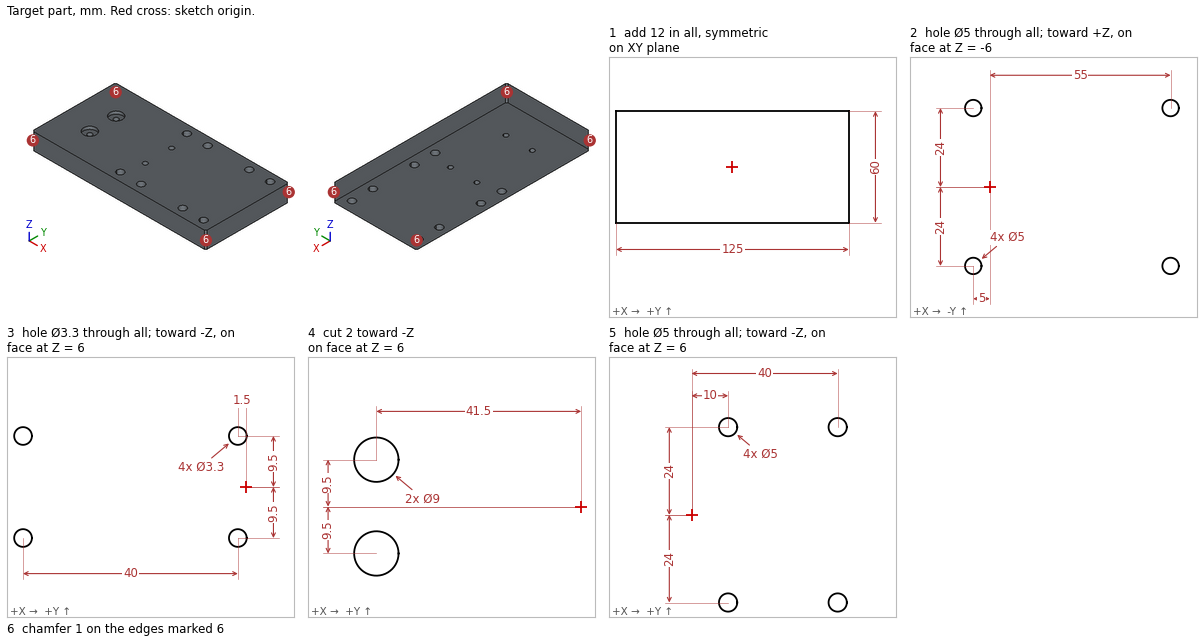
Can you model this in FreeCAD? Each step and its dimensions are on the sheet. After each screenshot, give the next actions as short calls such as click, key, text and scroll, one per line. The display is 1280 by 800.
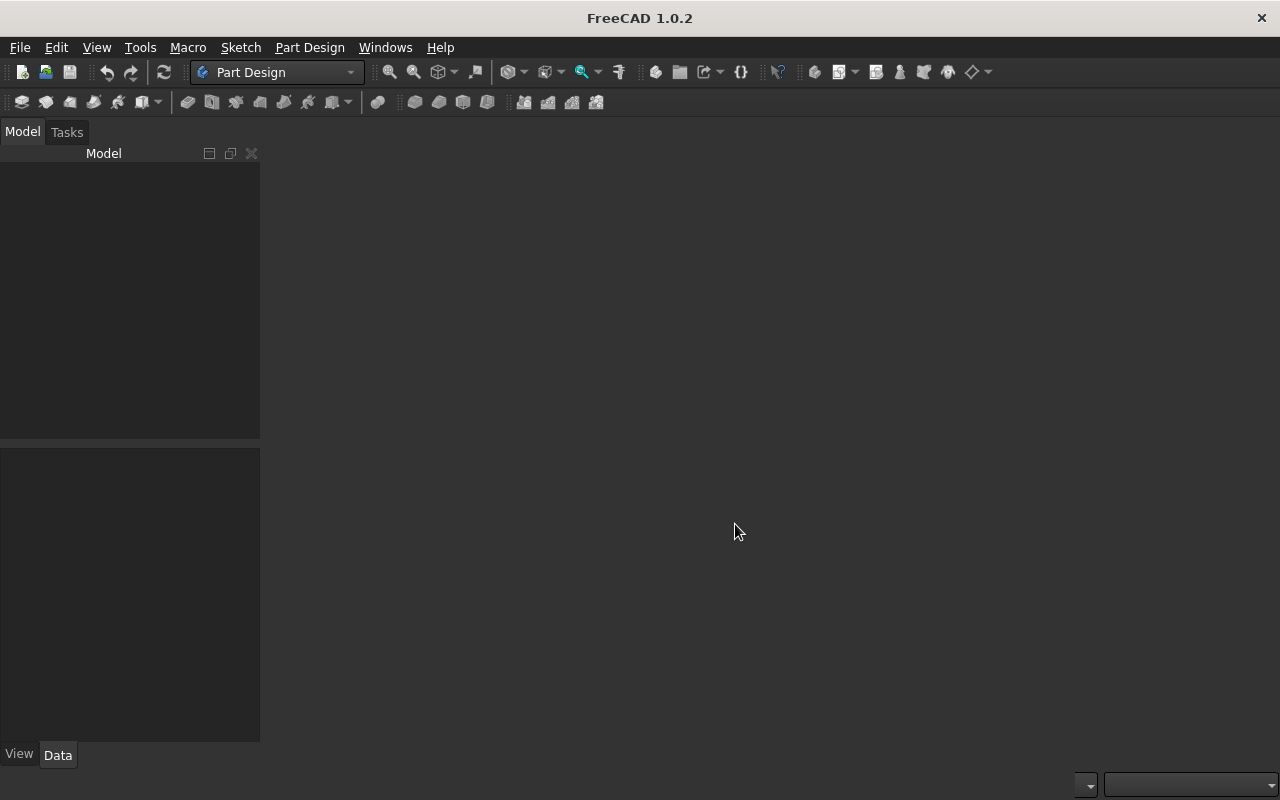
click(22, 72)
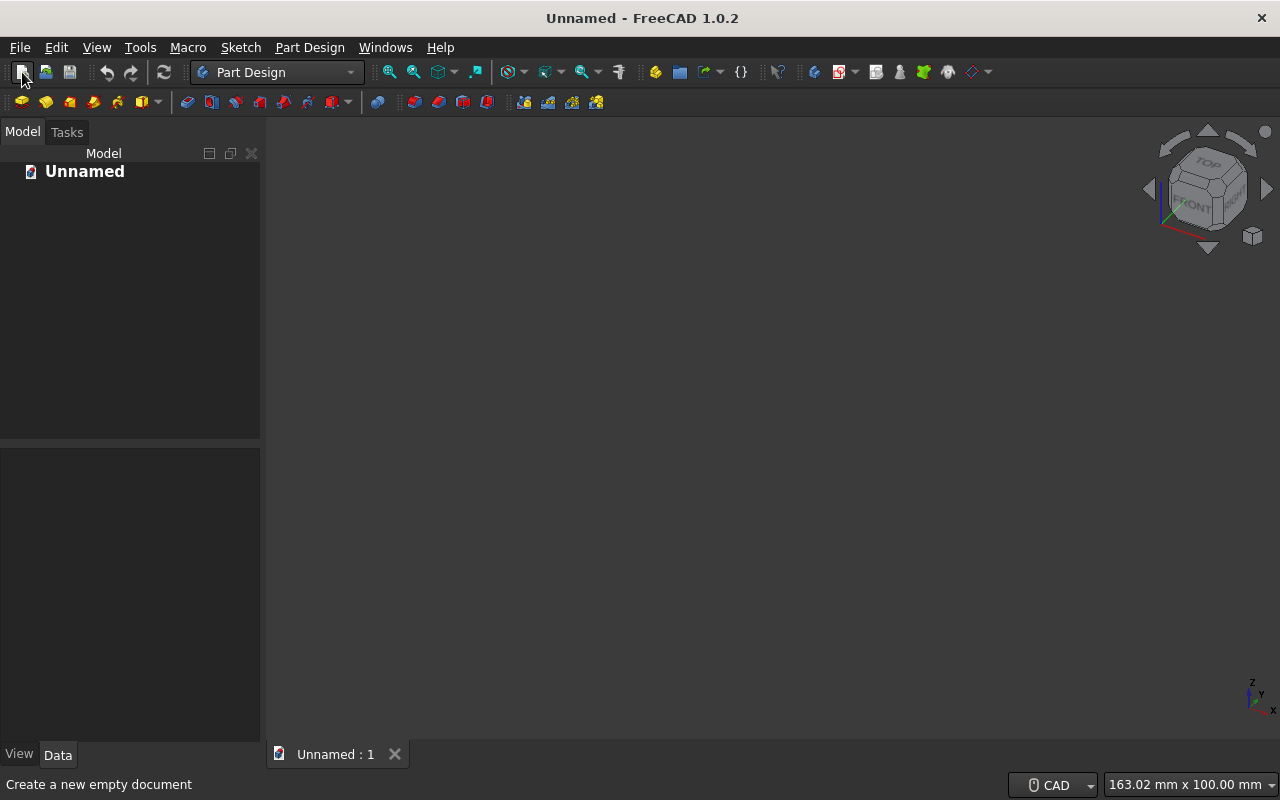
click(840, 72)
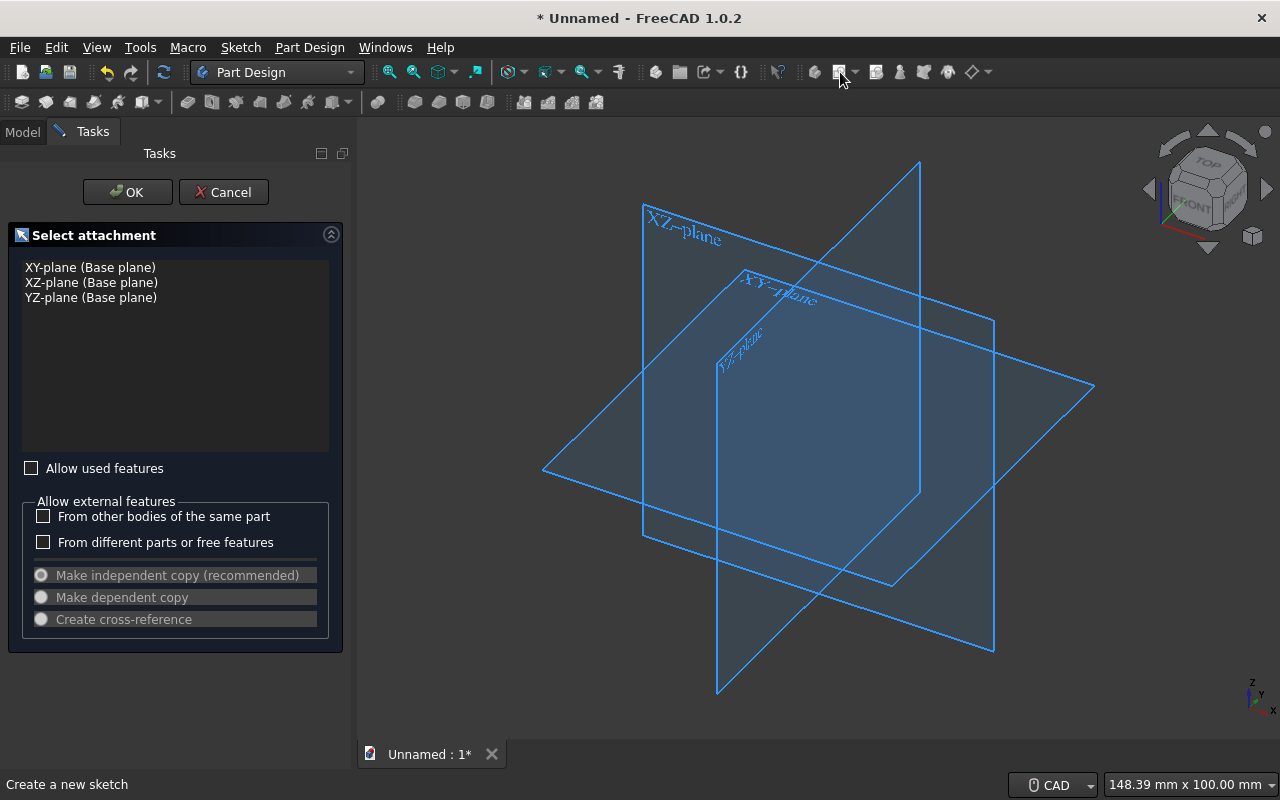
click(82, 268)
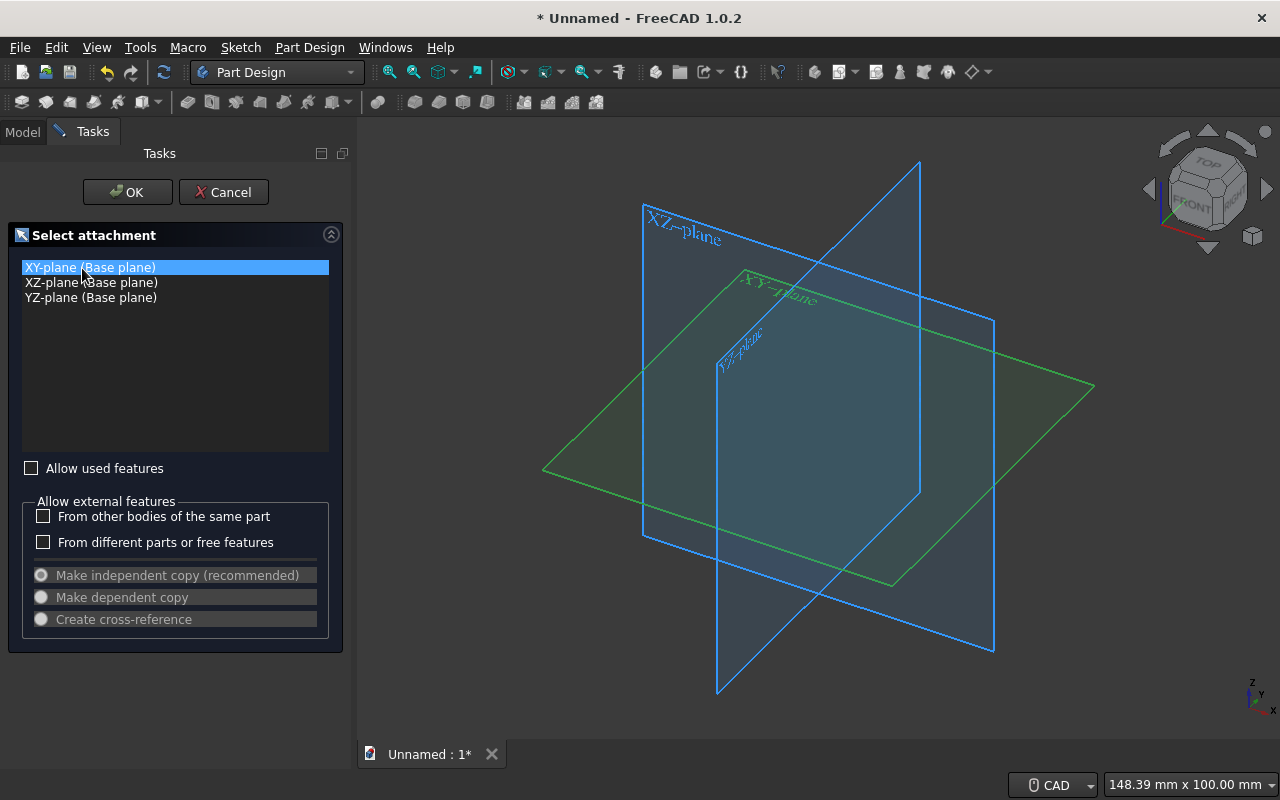
click(128, 192)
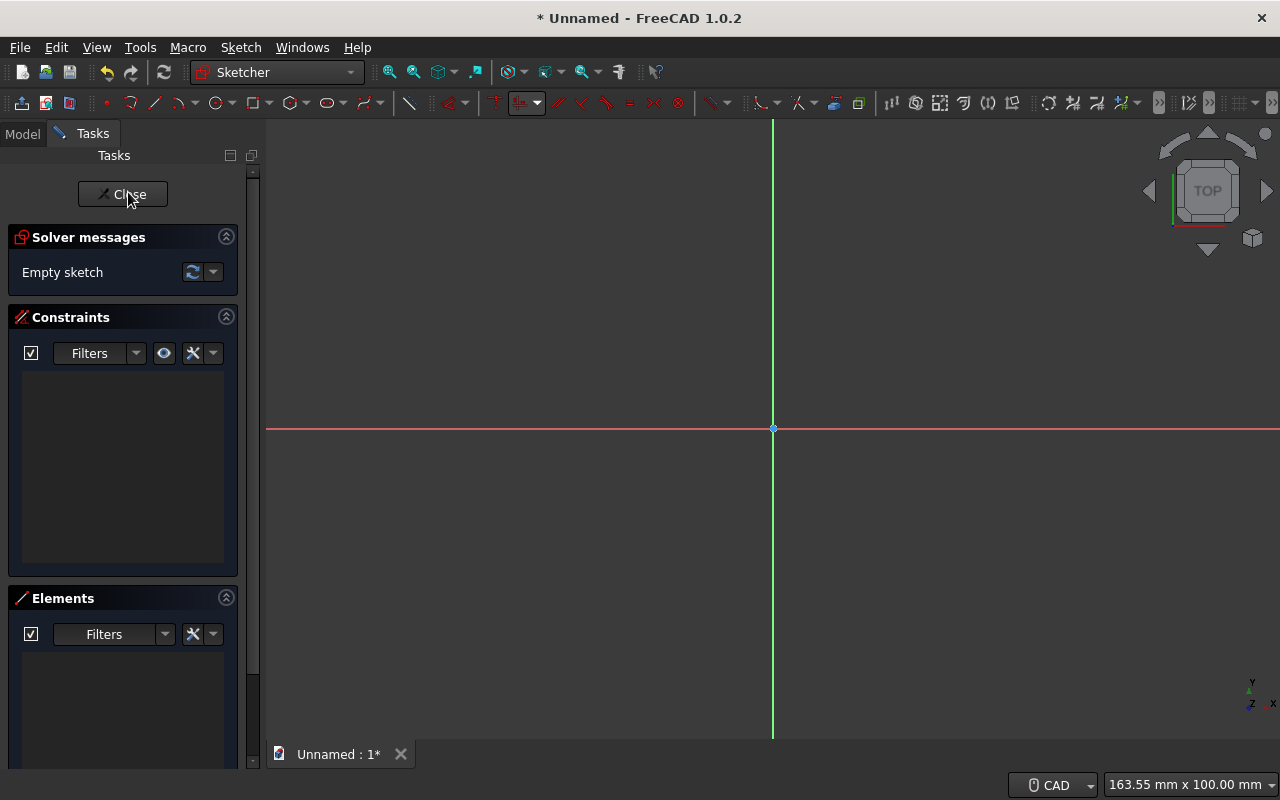
scroll(395, 429, down, 1)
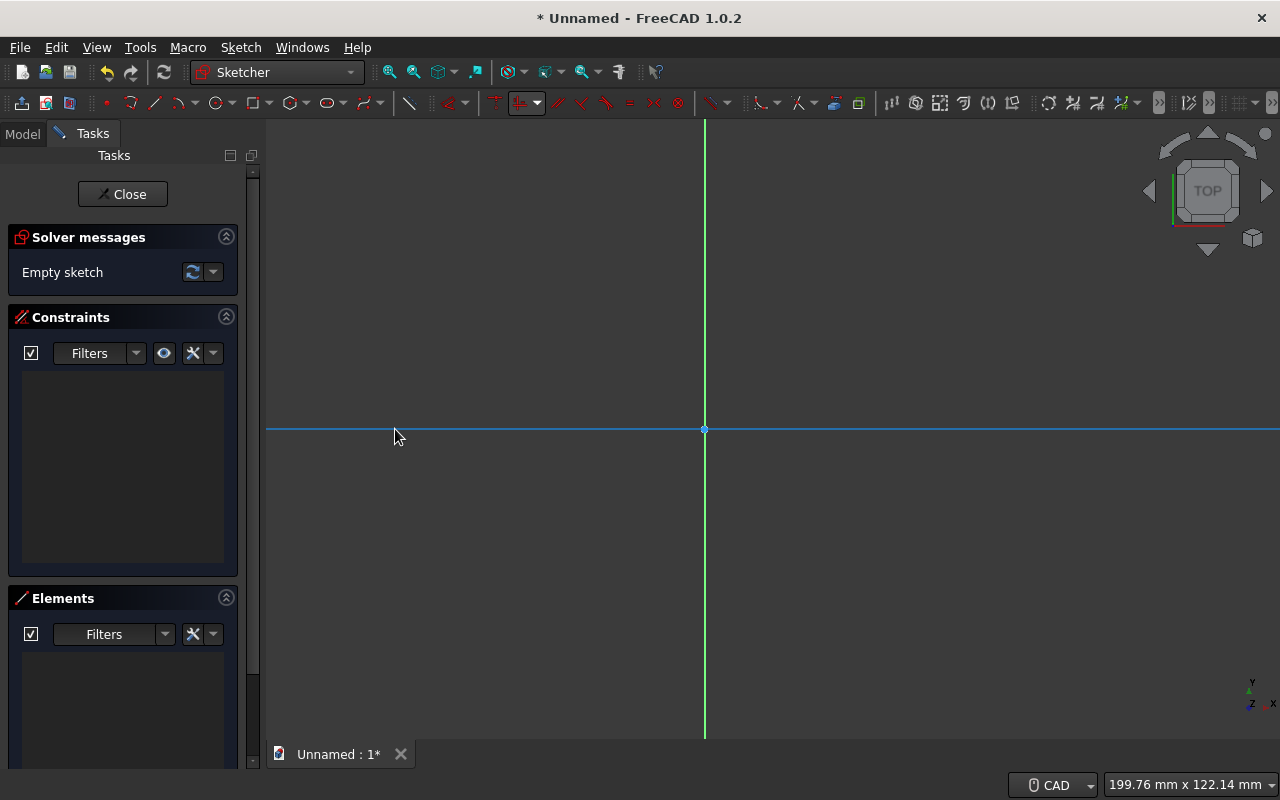
key(g)
key(v)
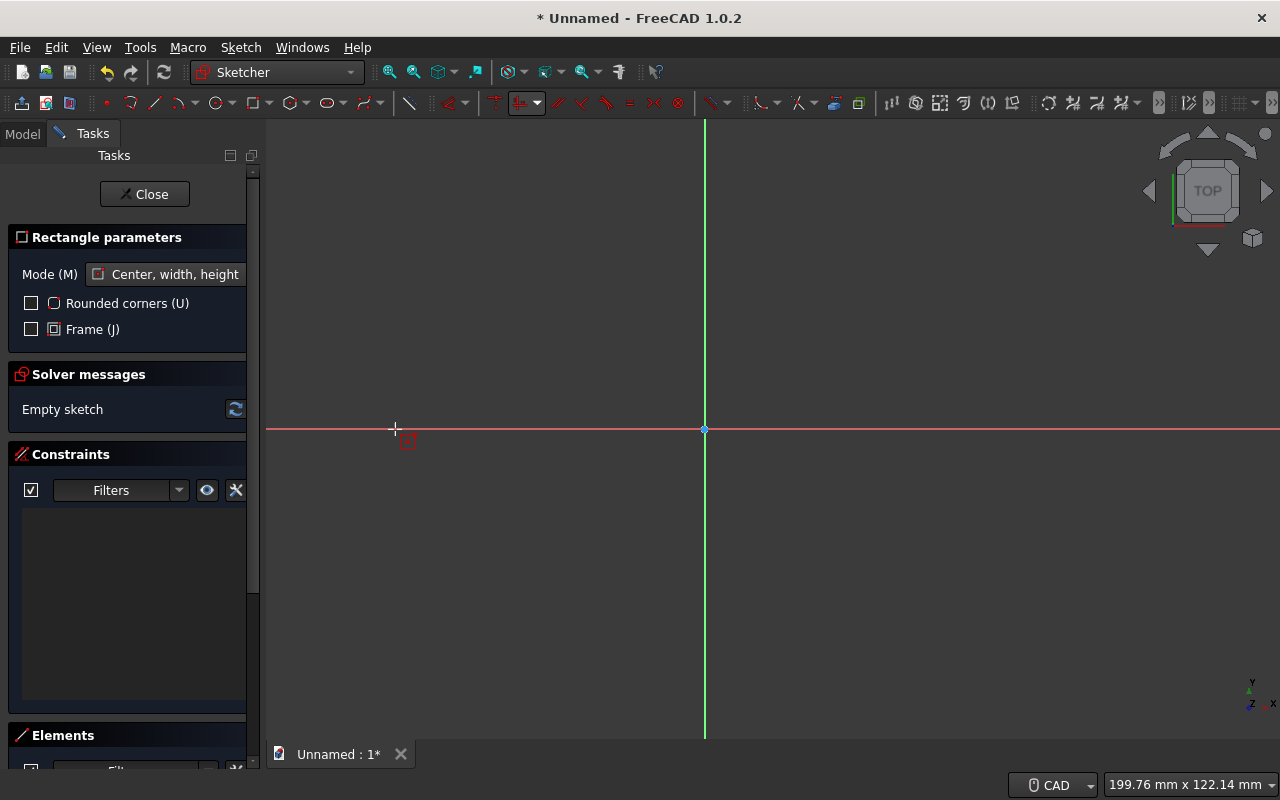
click(705, 429)
click(1022, 277)
key(Escape)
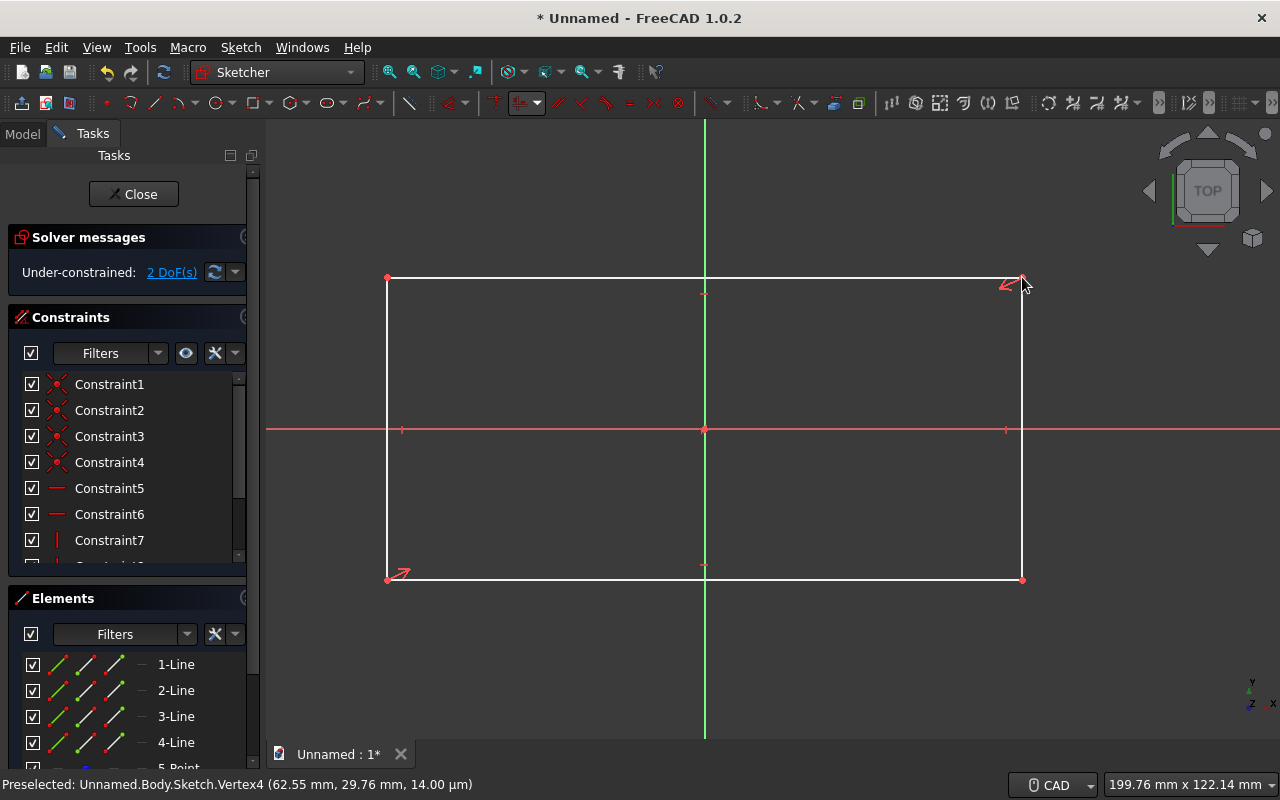
click(1022, 490)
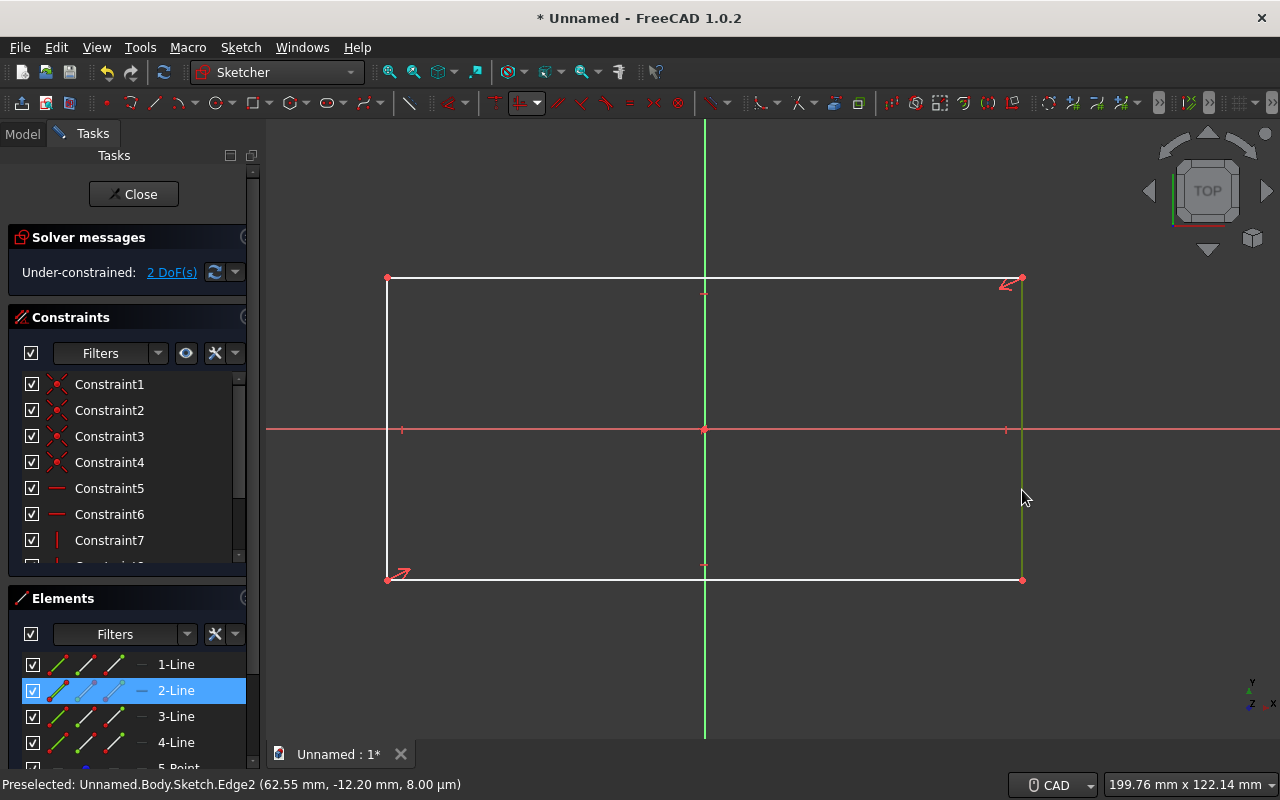
key(i)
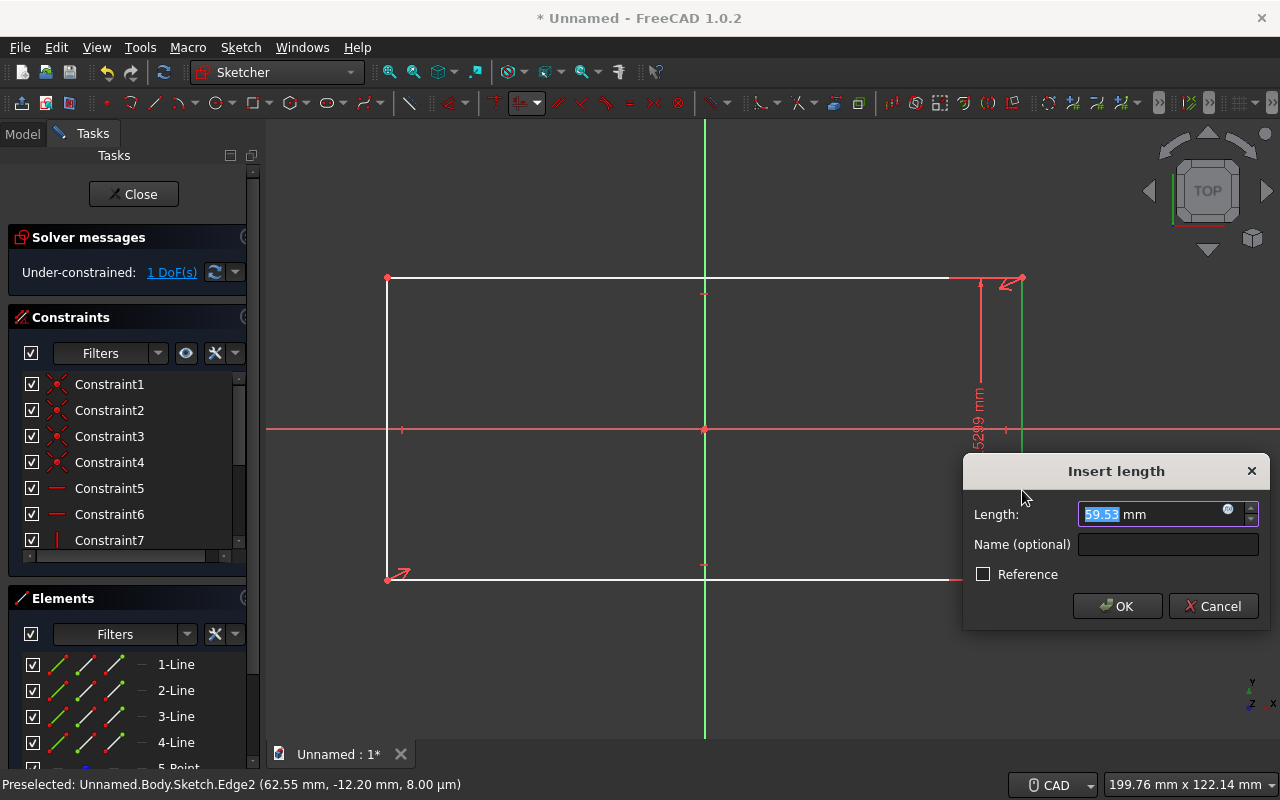
text(60)
key(Return)